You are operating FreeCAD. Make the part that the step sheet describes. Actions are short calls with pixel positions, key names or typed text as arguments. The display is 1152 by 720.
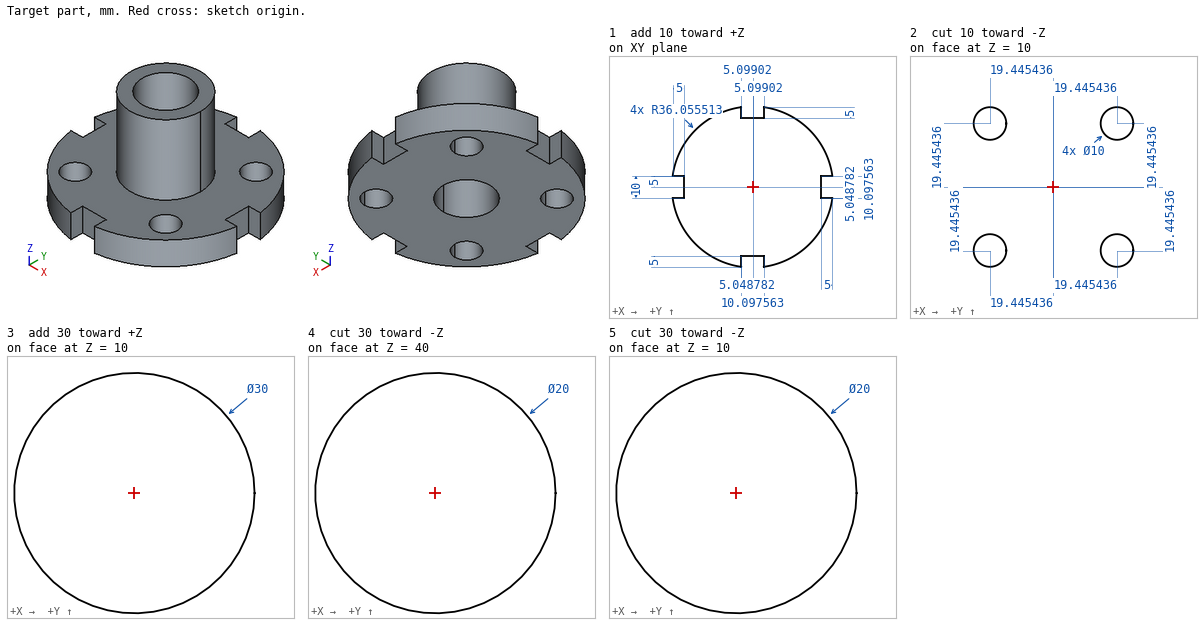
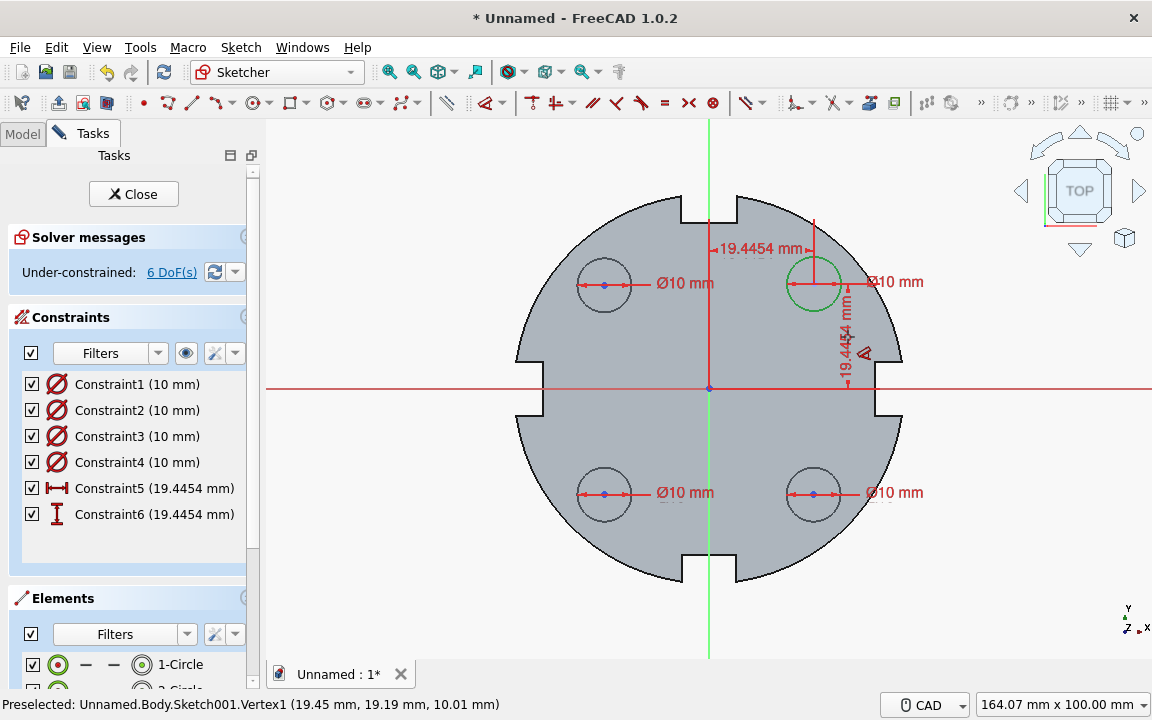
click(814, 495)
click(761, 529)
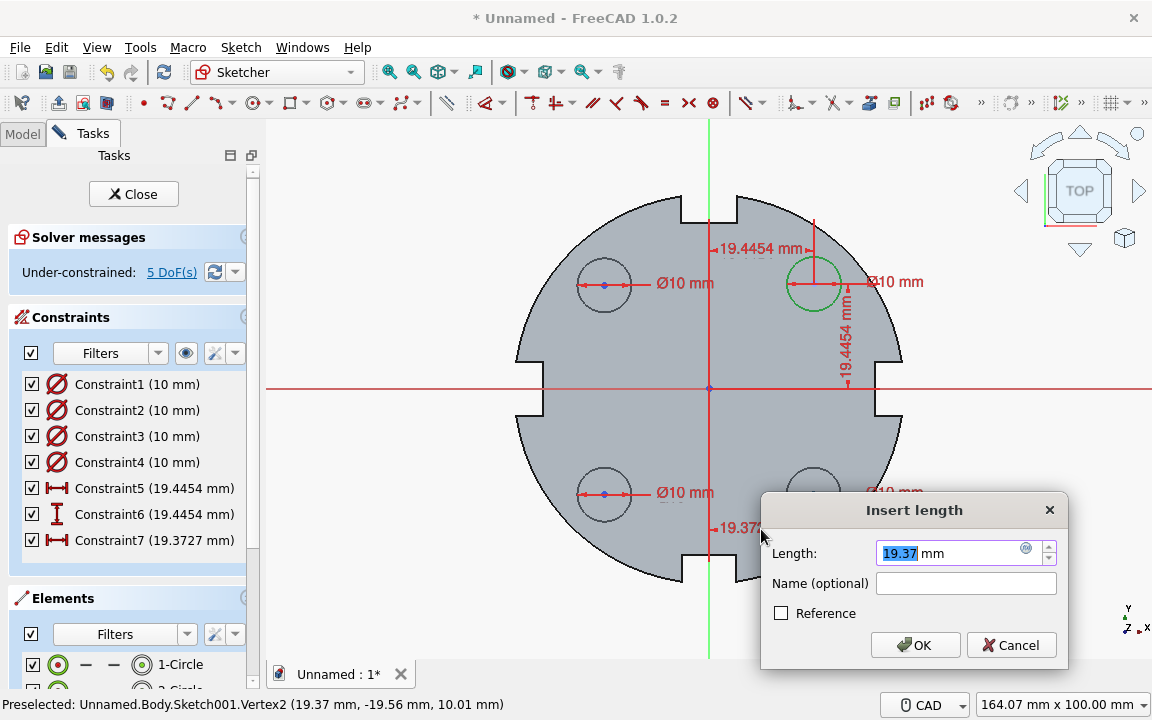
text(19.445436)
key(Return)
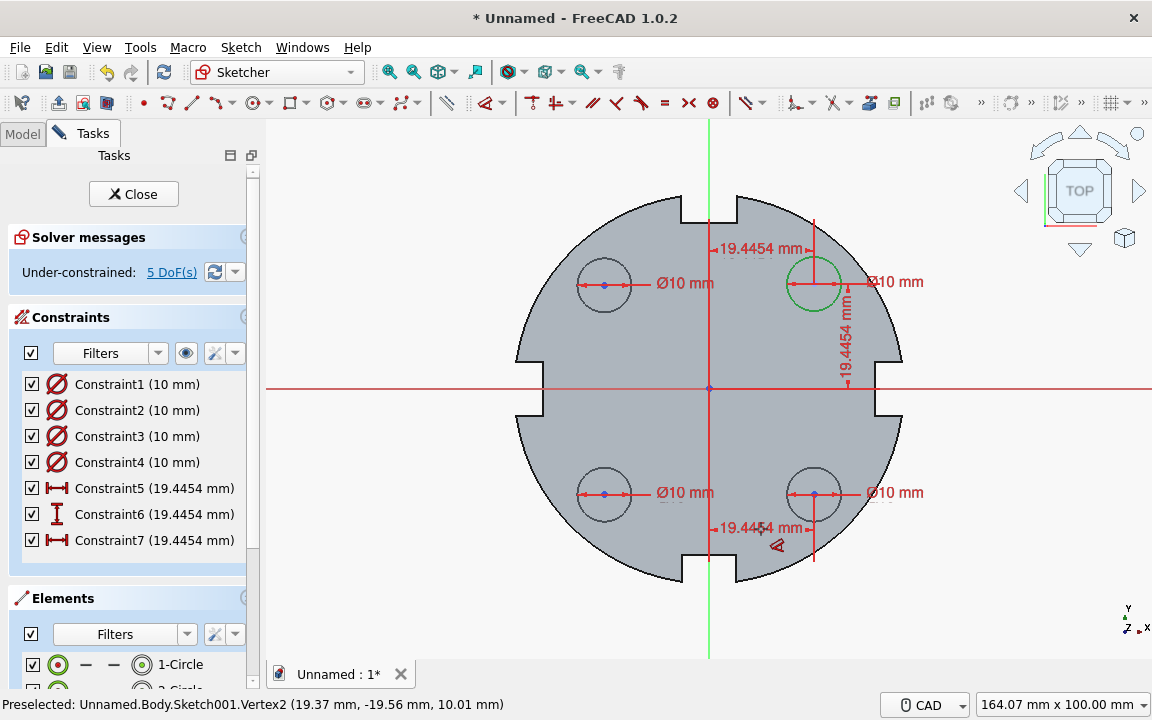
click(814, 495)
click(848, 442)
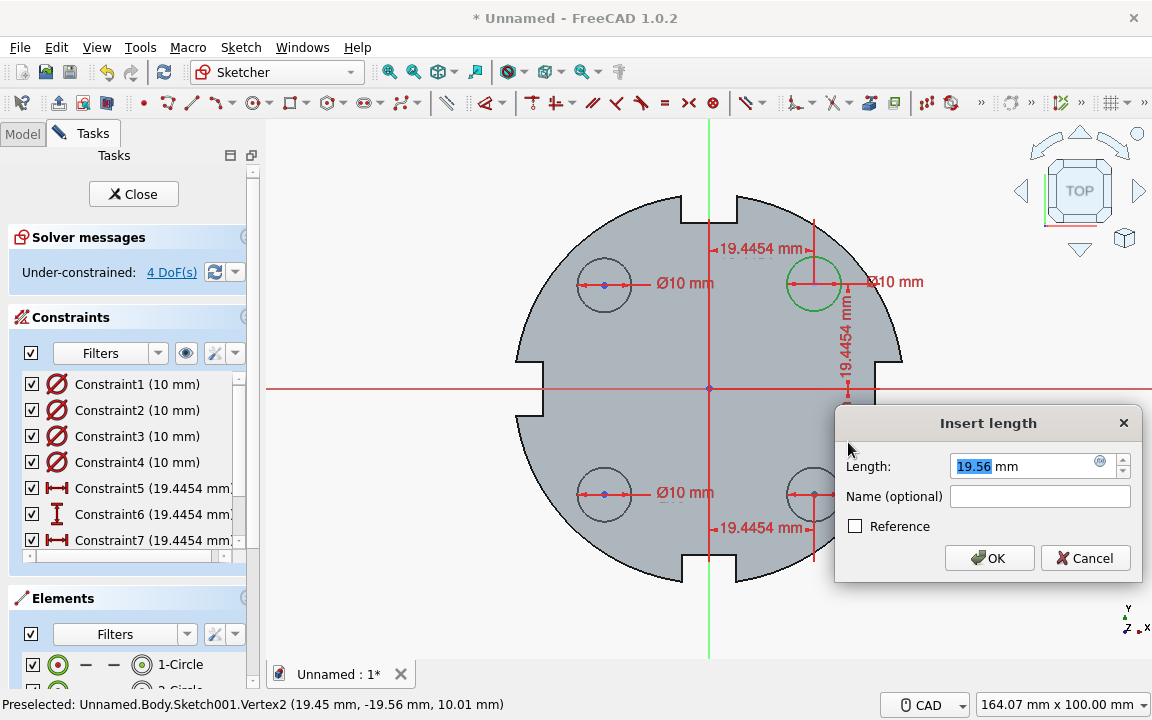
text(19.445436)
key(Return)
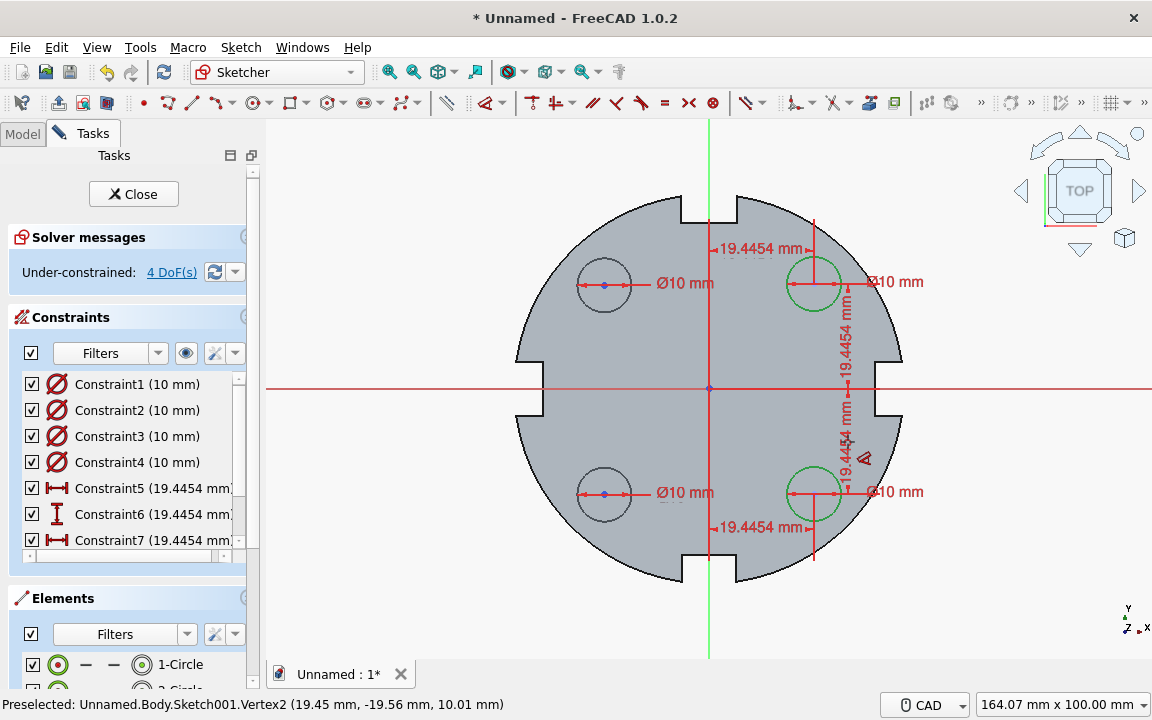
click(604, 495)
click(657, 529)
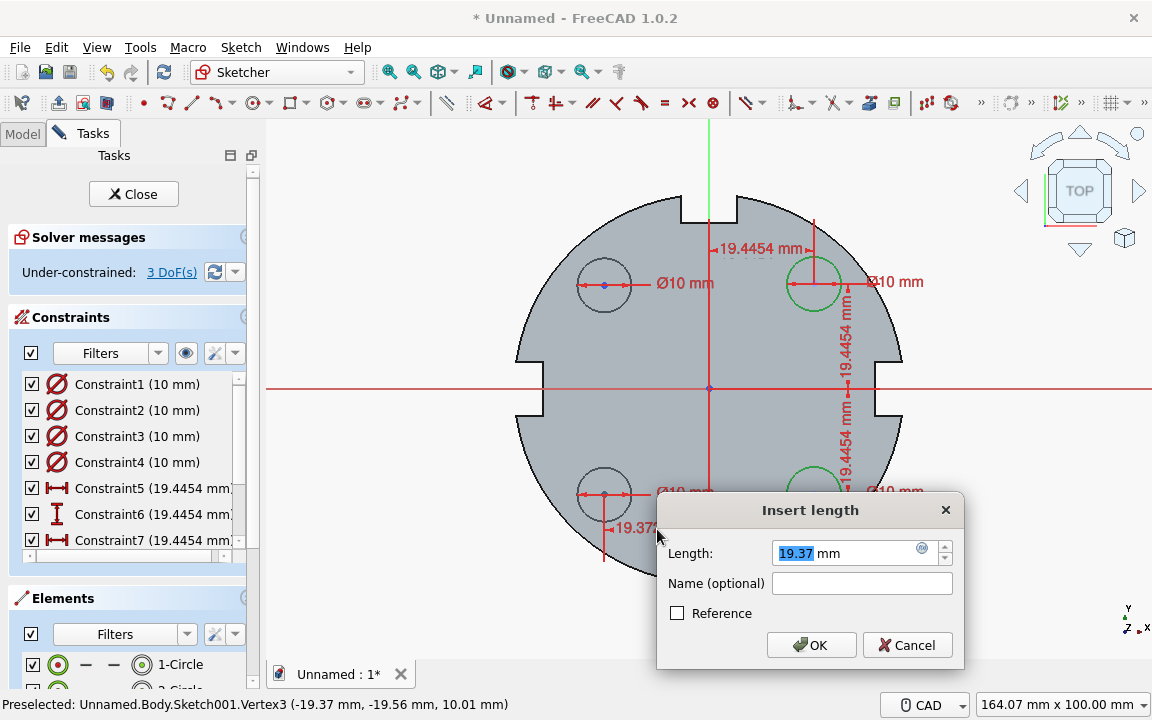
text(19.445436)
key(Return)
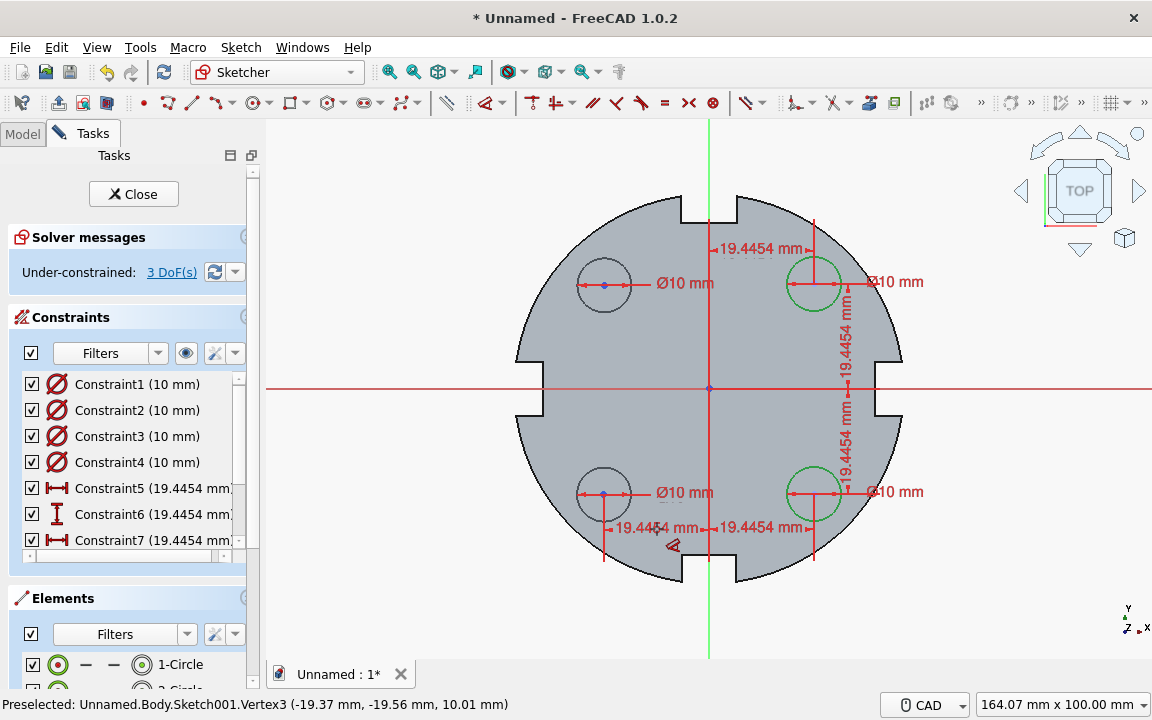
click(604, 495)
click(570, 442)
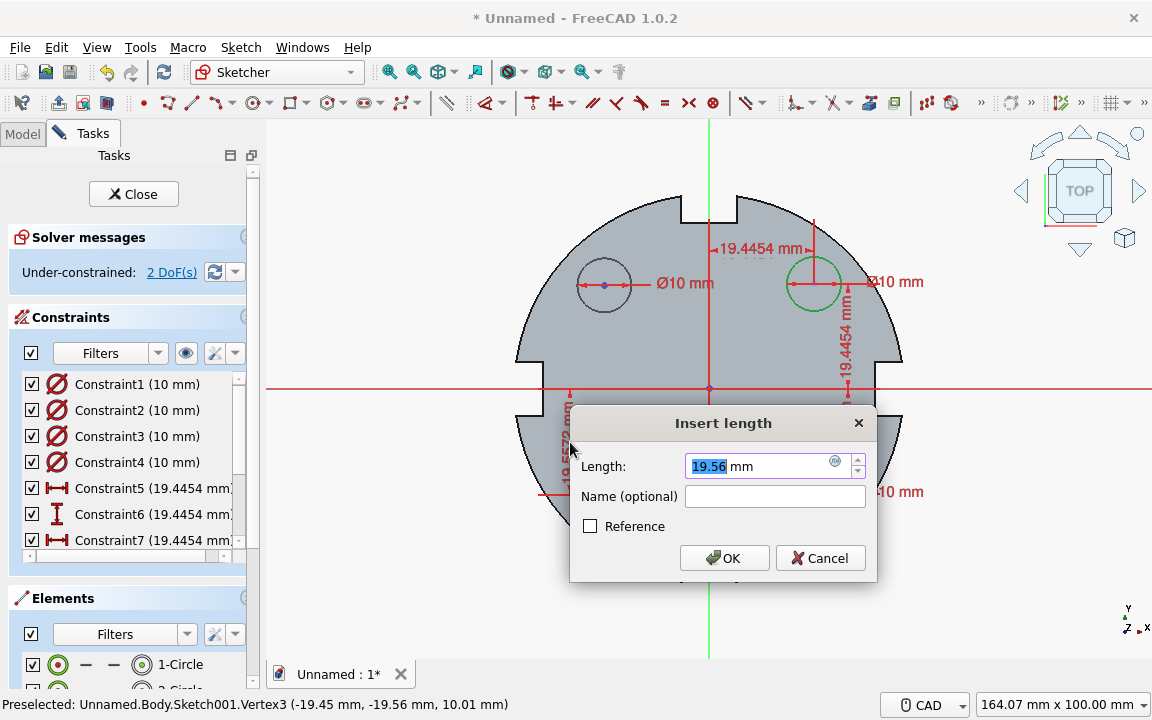
text(19.445436)
key(Return)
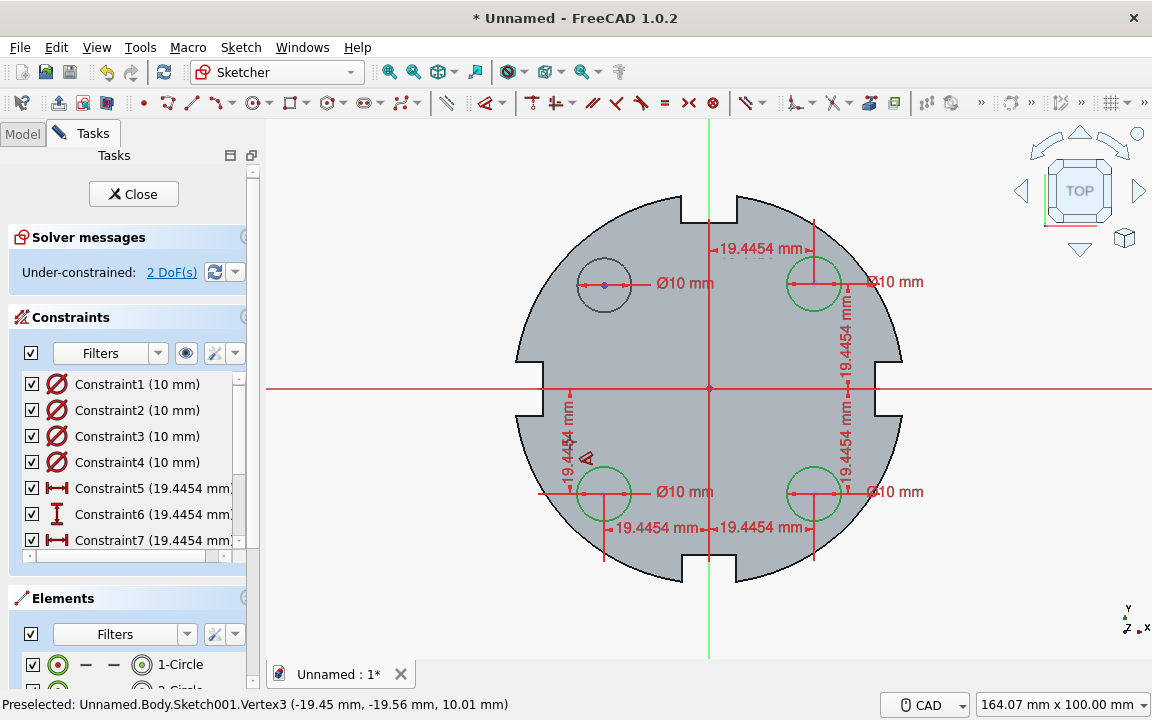
click(604, 285)
click(657, 251)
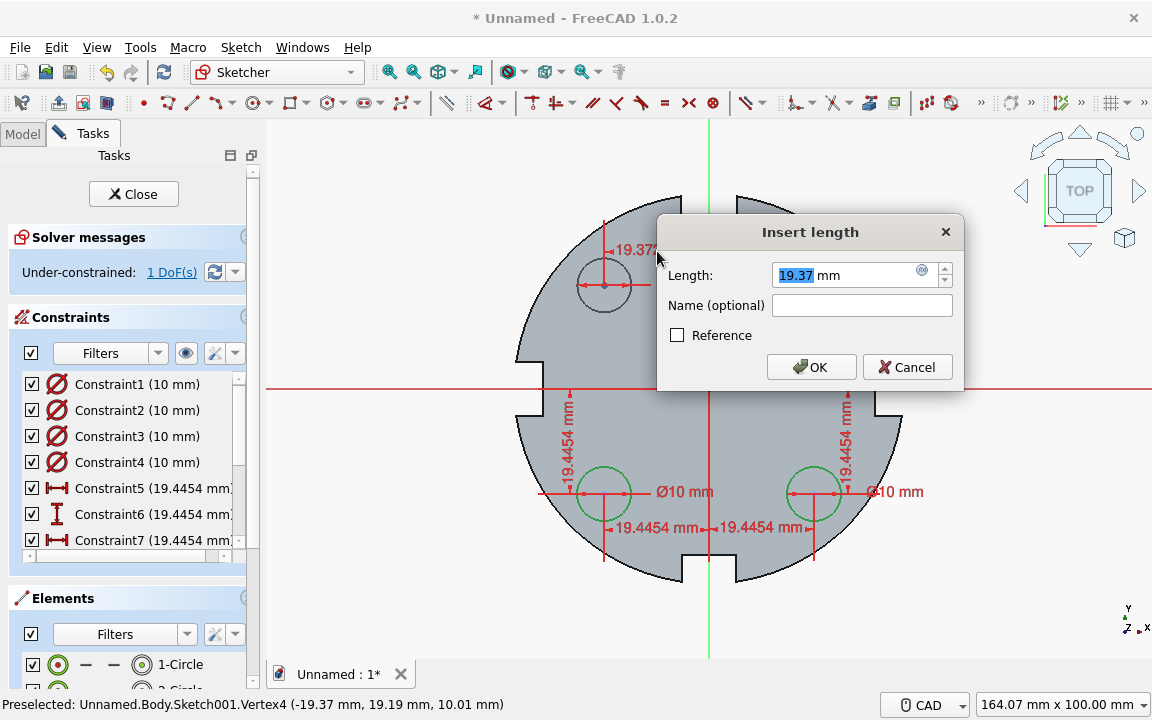
text(19.445436)
key(Return)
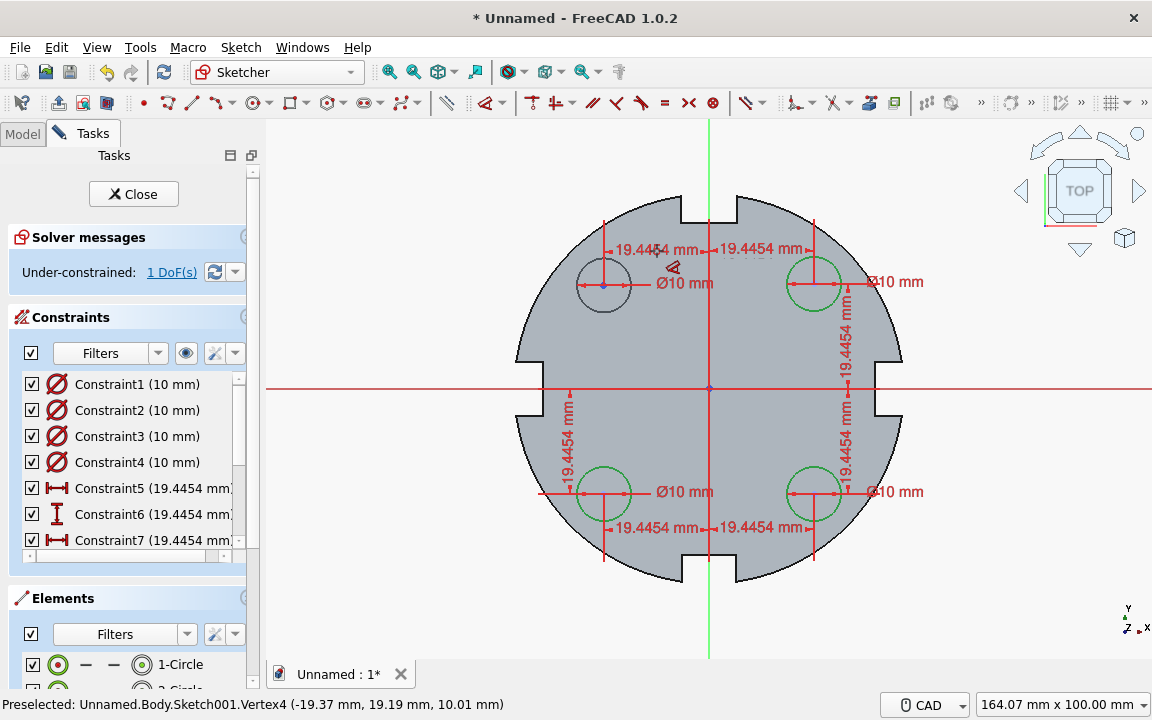
click(604, 285)
click(570, 337)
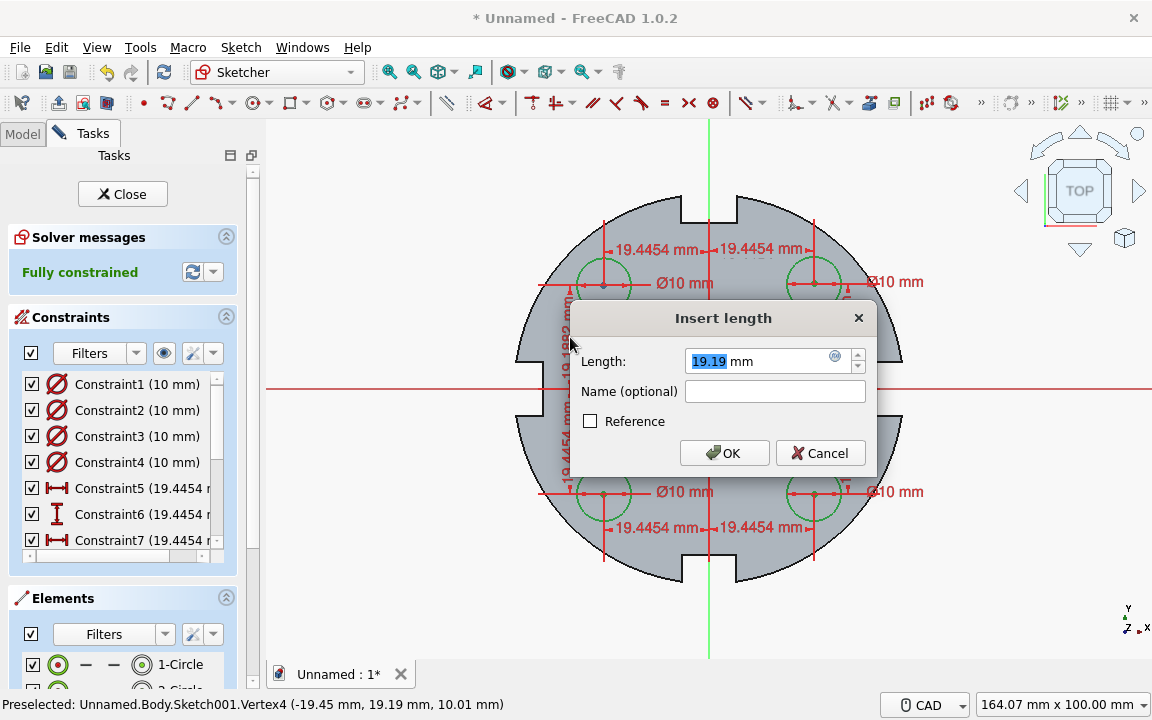
text(19.445436)
key(Return)
key(Escape)